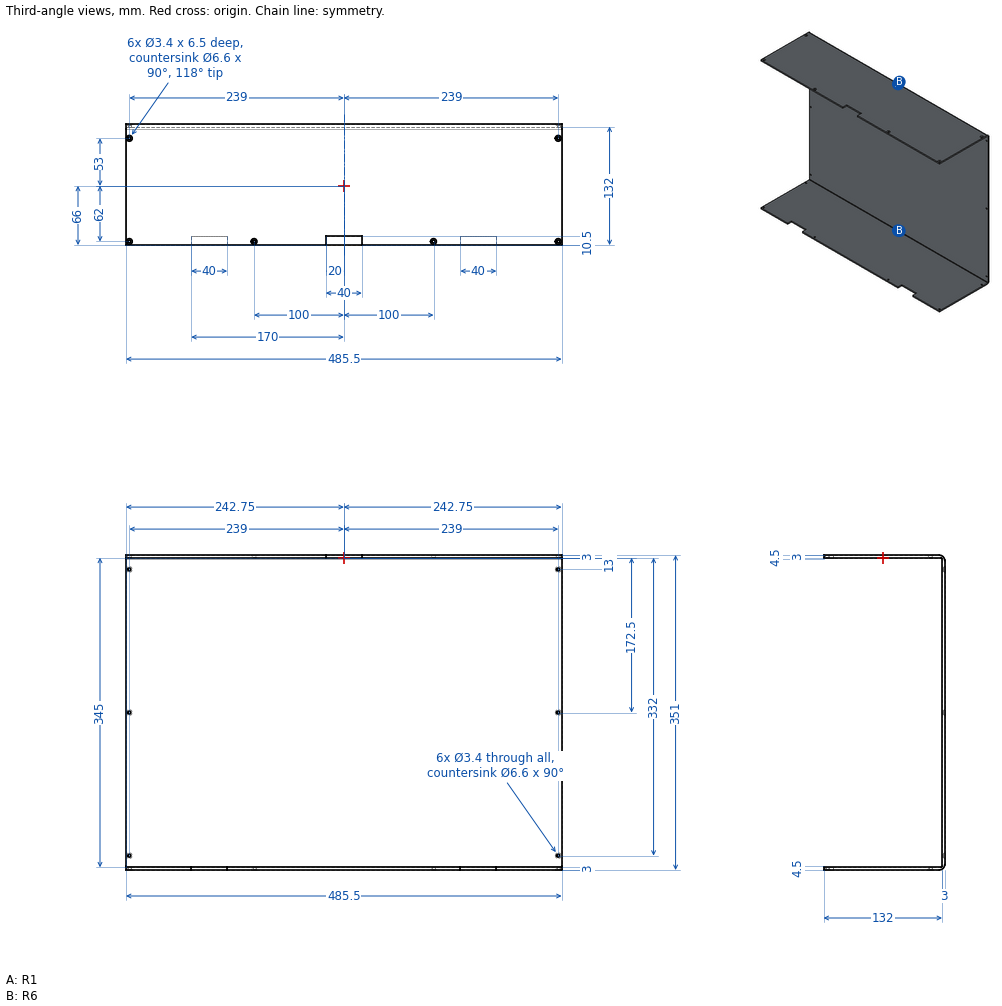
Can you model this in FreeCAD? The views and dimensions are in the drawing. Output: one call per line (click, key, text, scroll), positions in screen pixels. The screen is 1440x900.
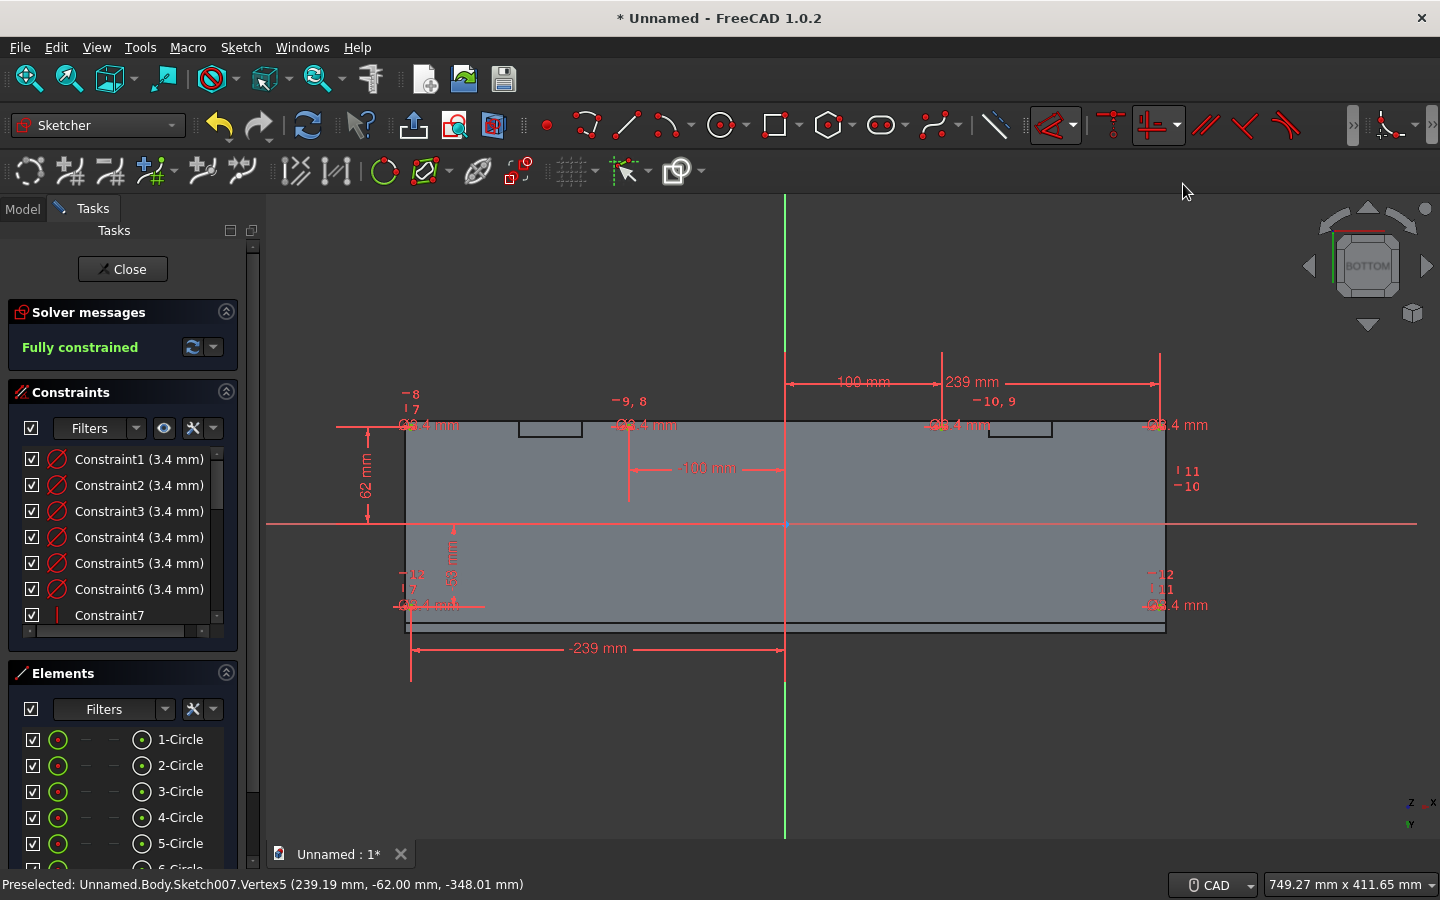
click(123, 269)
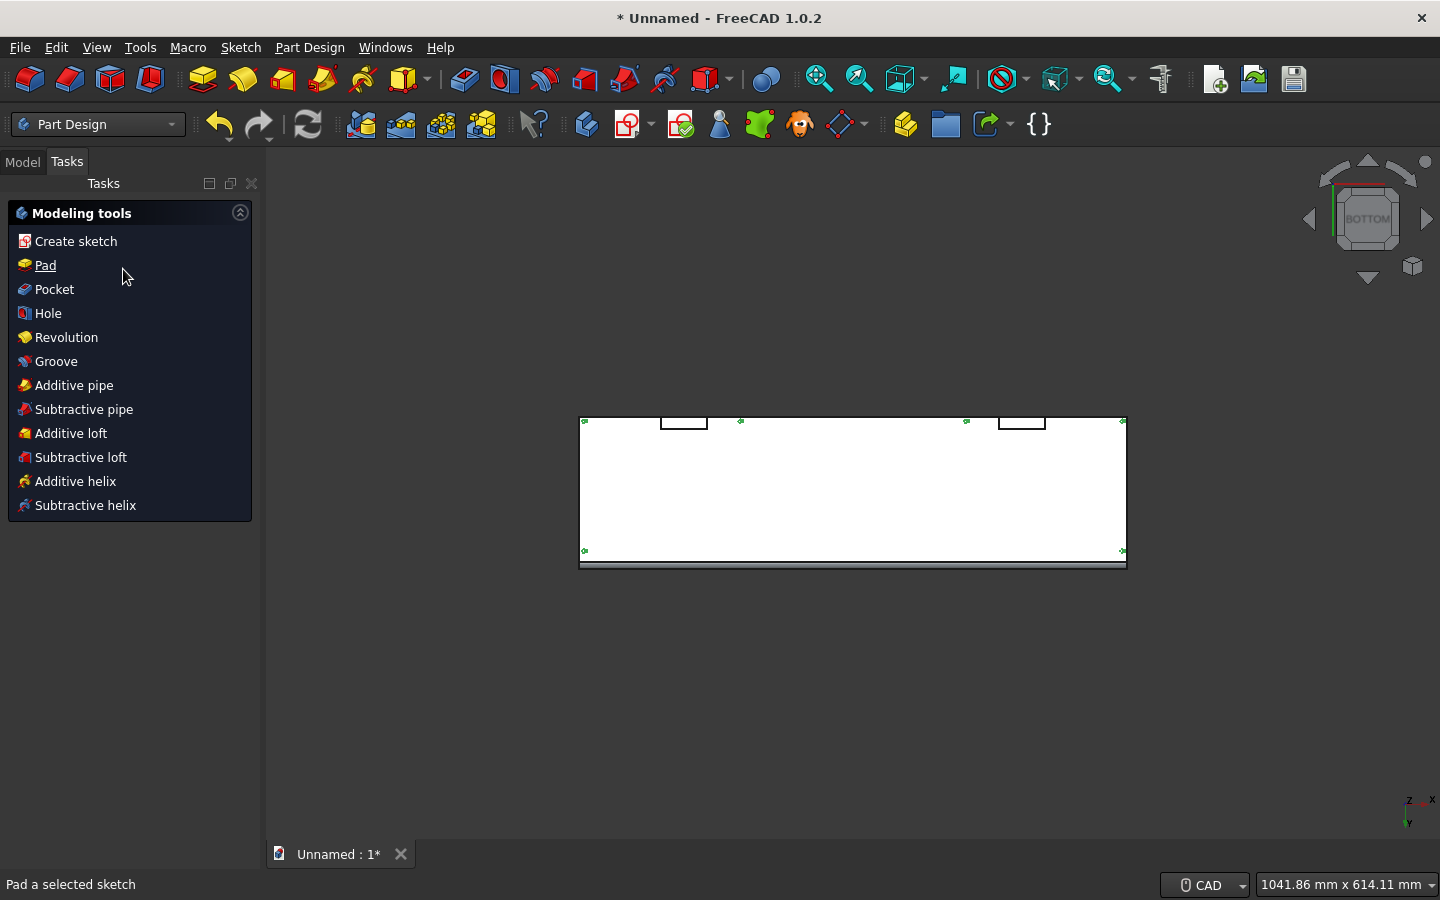
click(506, 80)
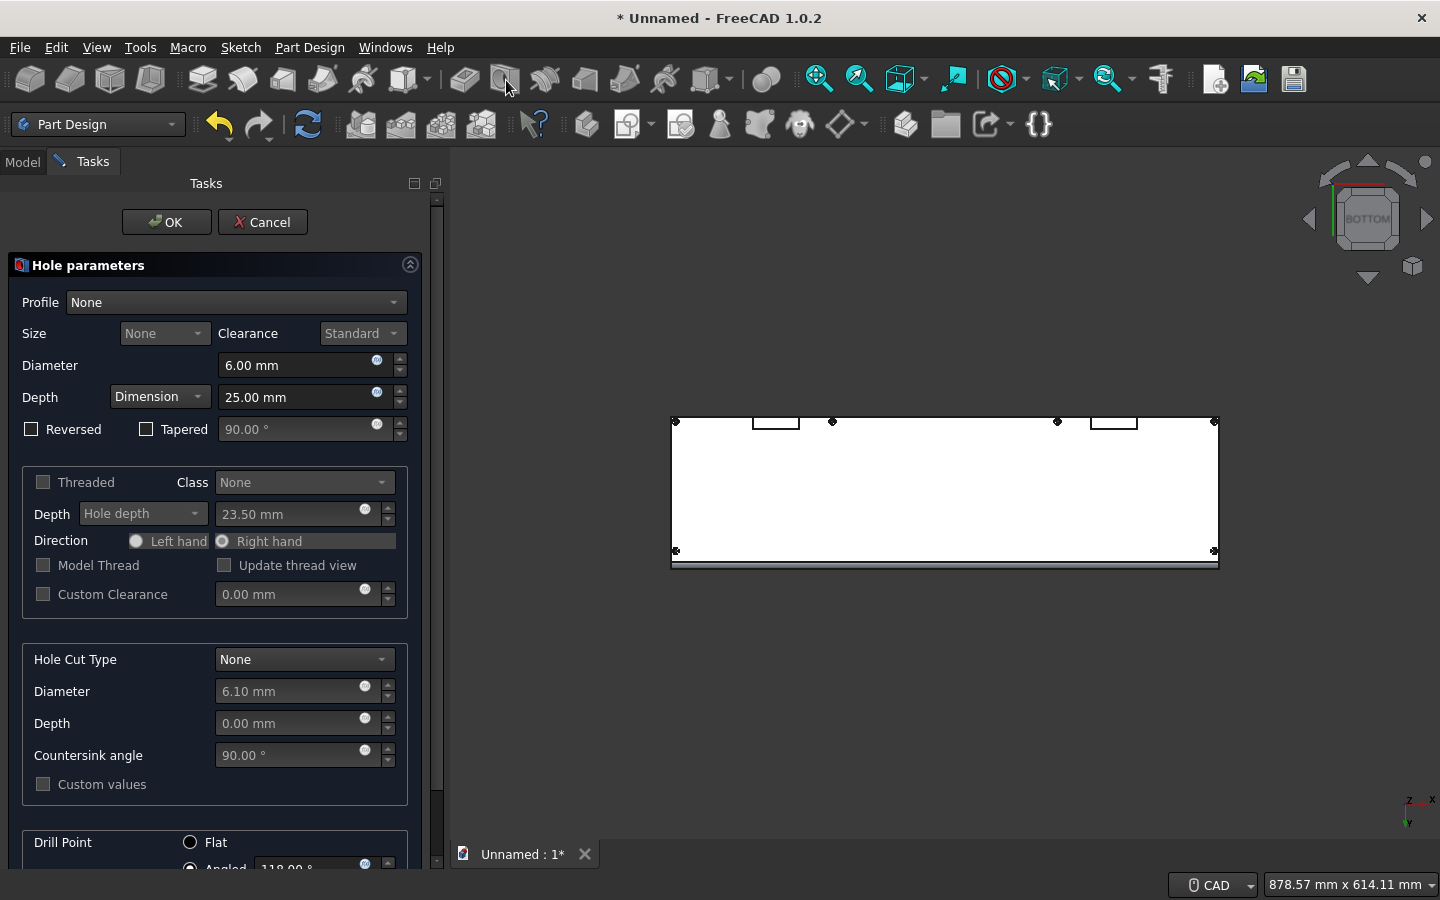
triple_click(305, 365)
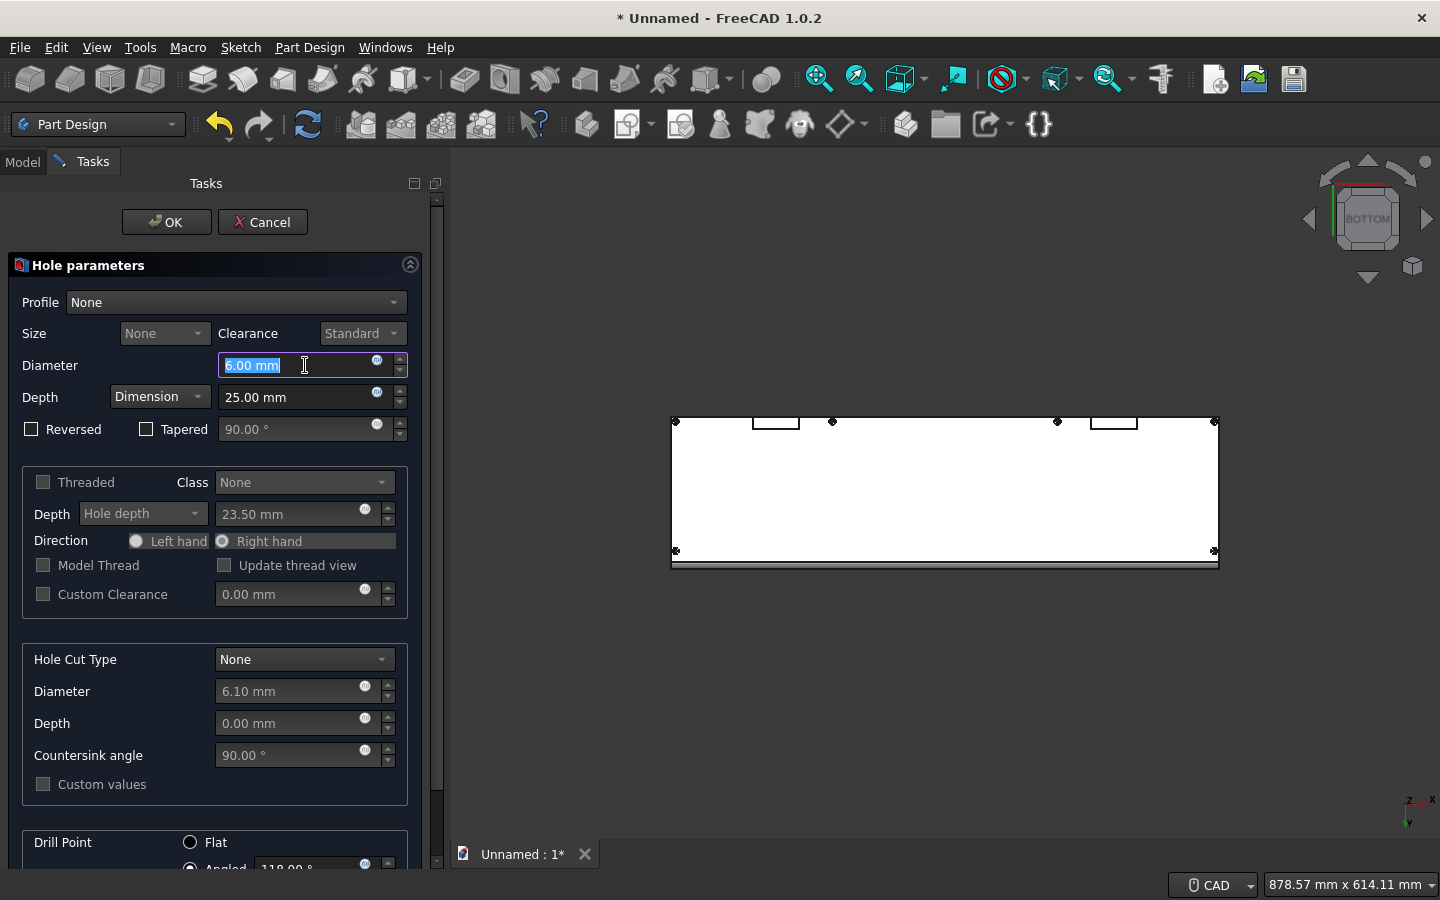
text(3.4)
key(Tab)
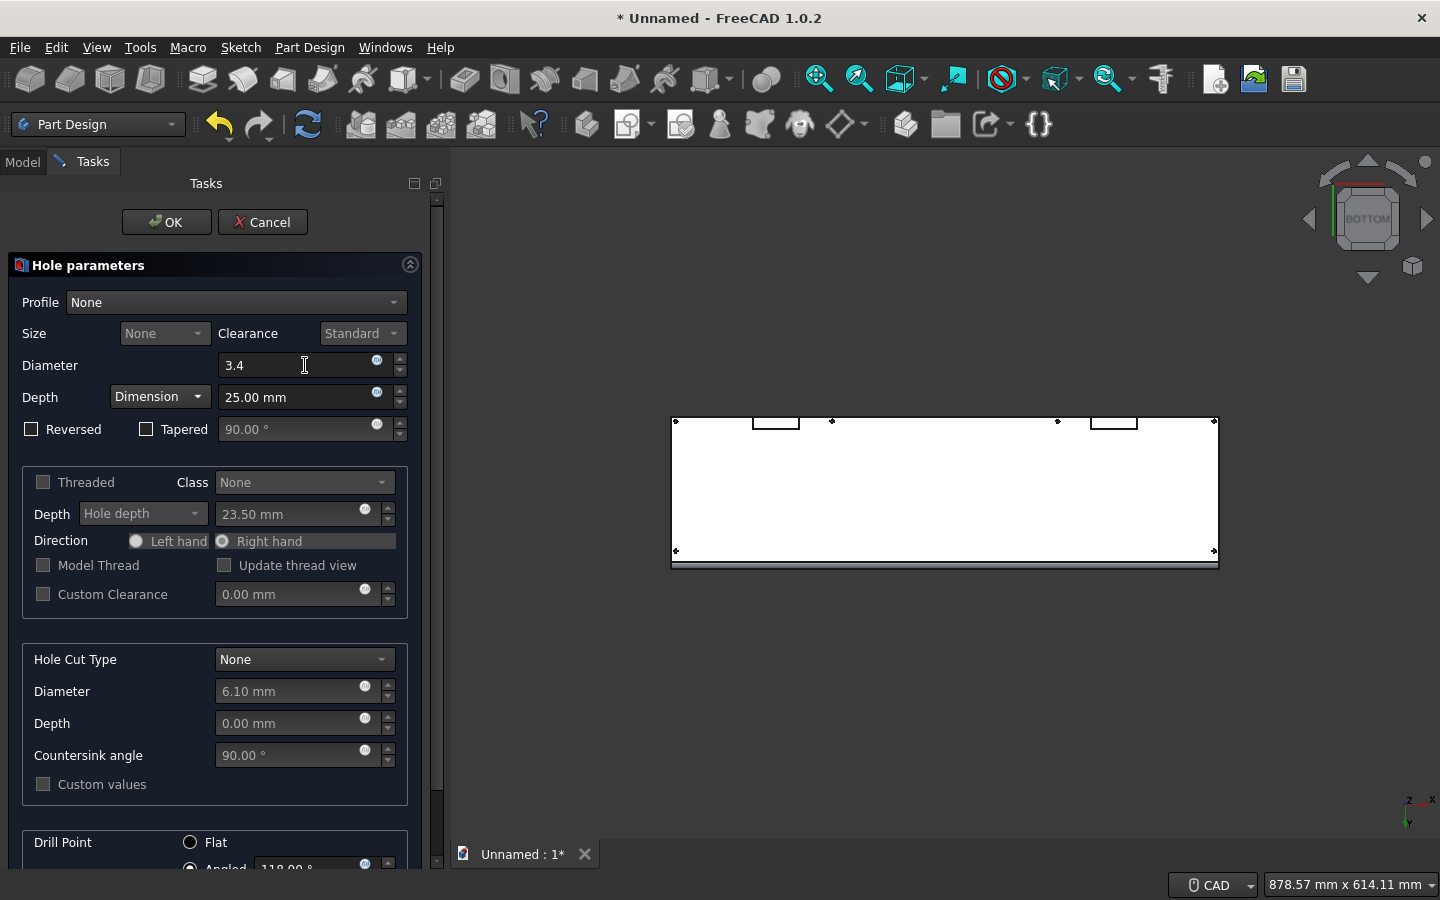
triple_click(305, 397)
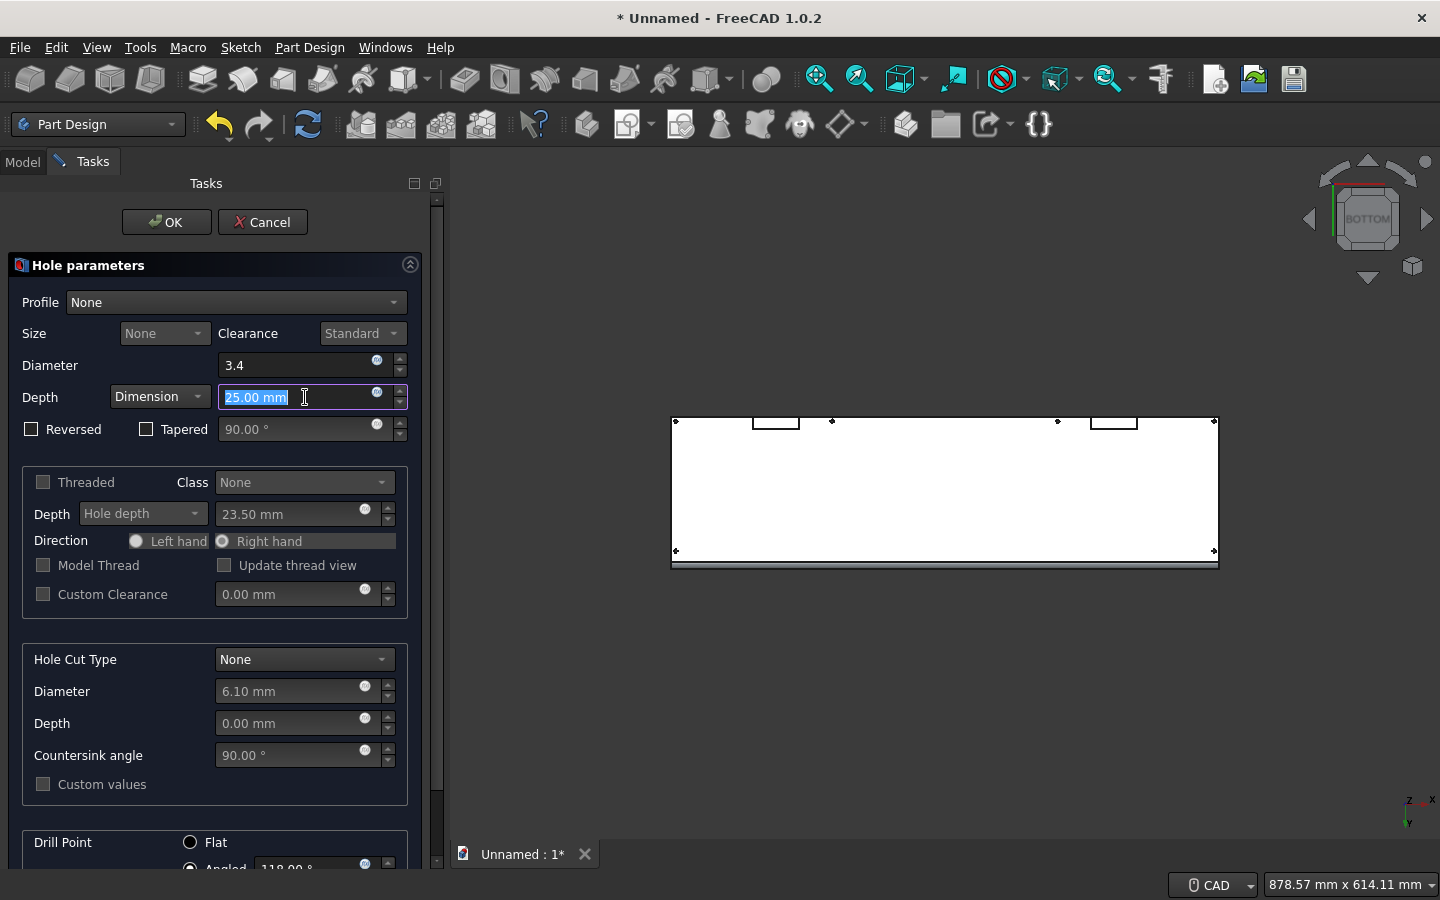
text(6.5)
key(Tab)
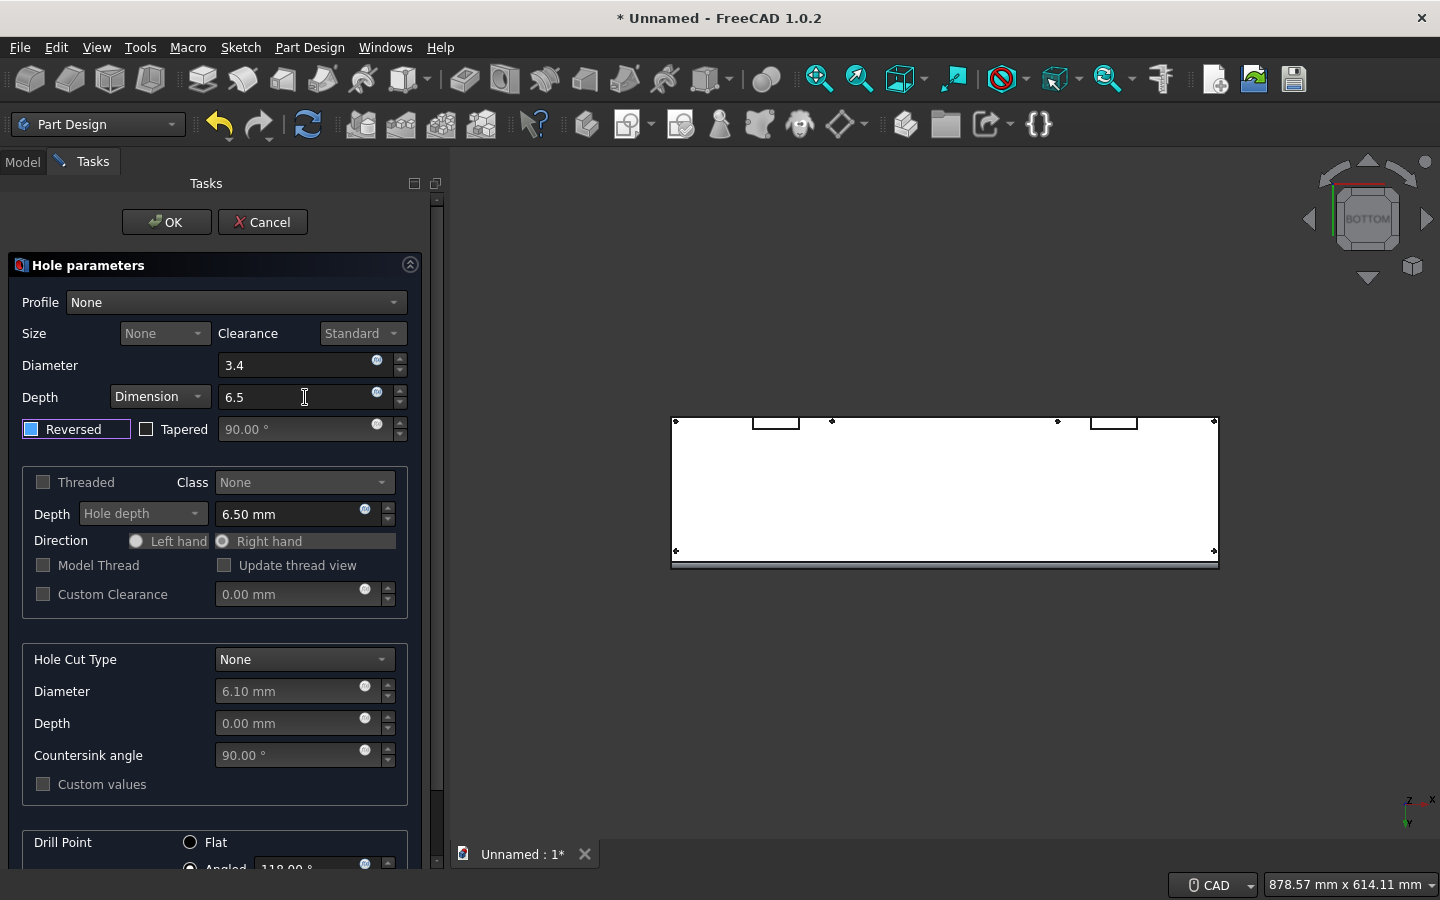
click(306, 660)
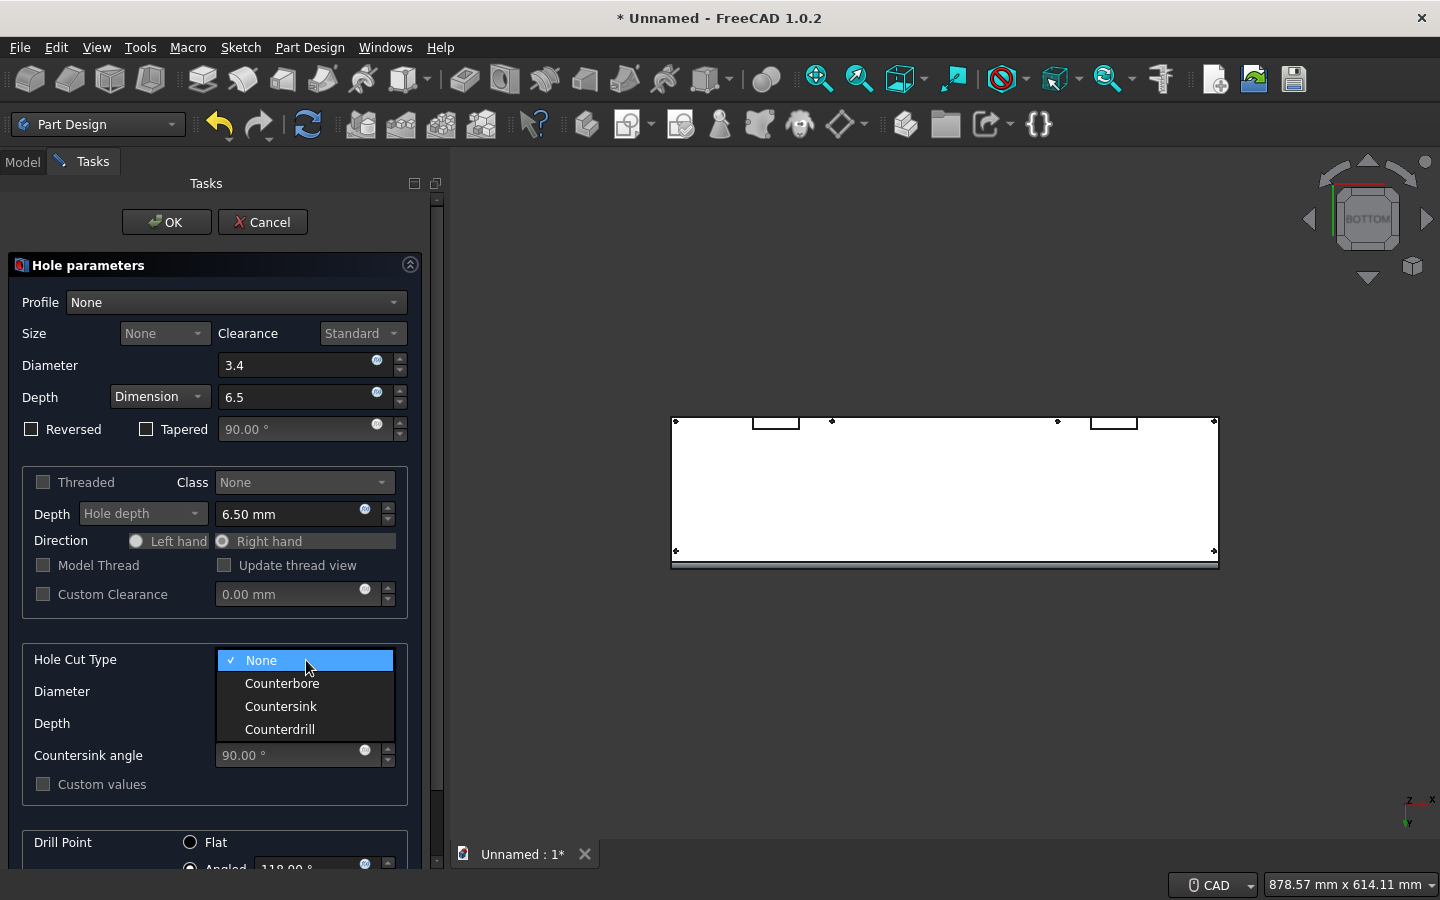
click(304, 706)